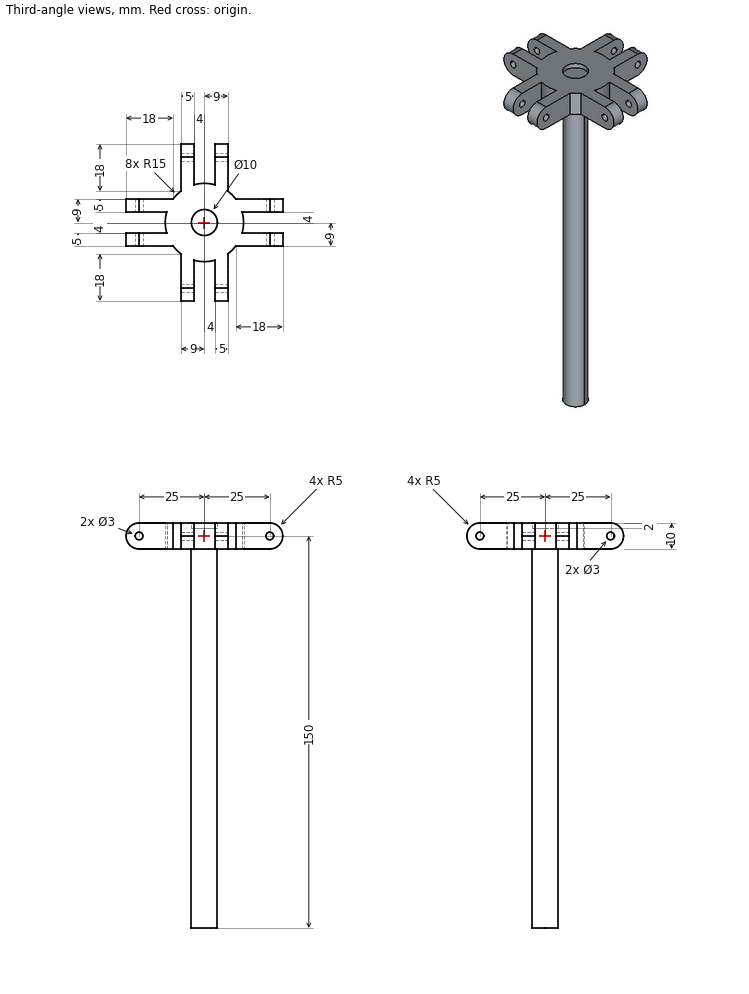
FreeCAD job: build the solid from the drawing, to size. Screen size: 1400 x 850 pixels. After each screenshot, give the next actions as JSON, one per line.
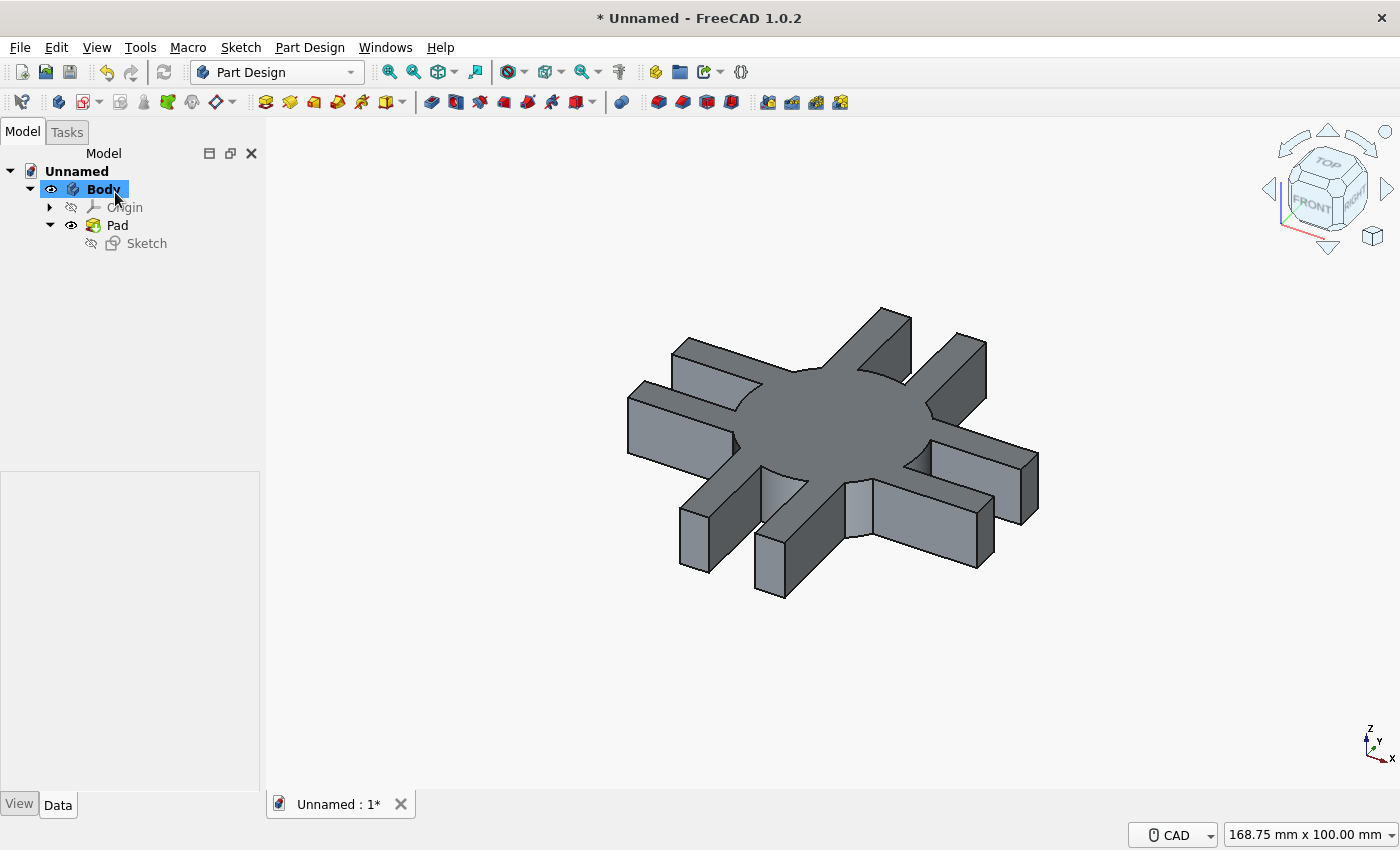
{"action": "left_click", "coordinate": [84, 102]}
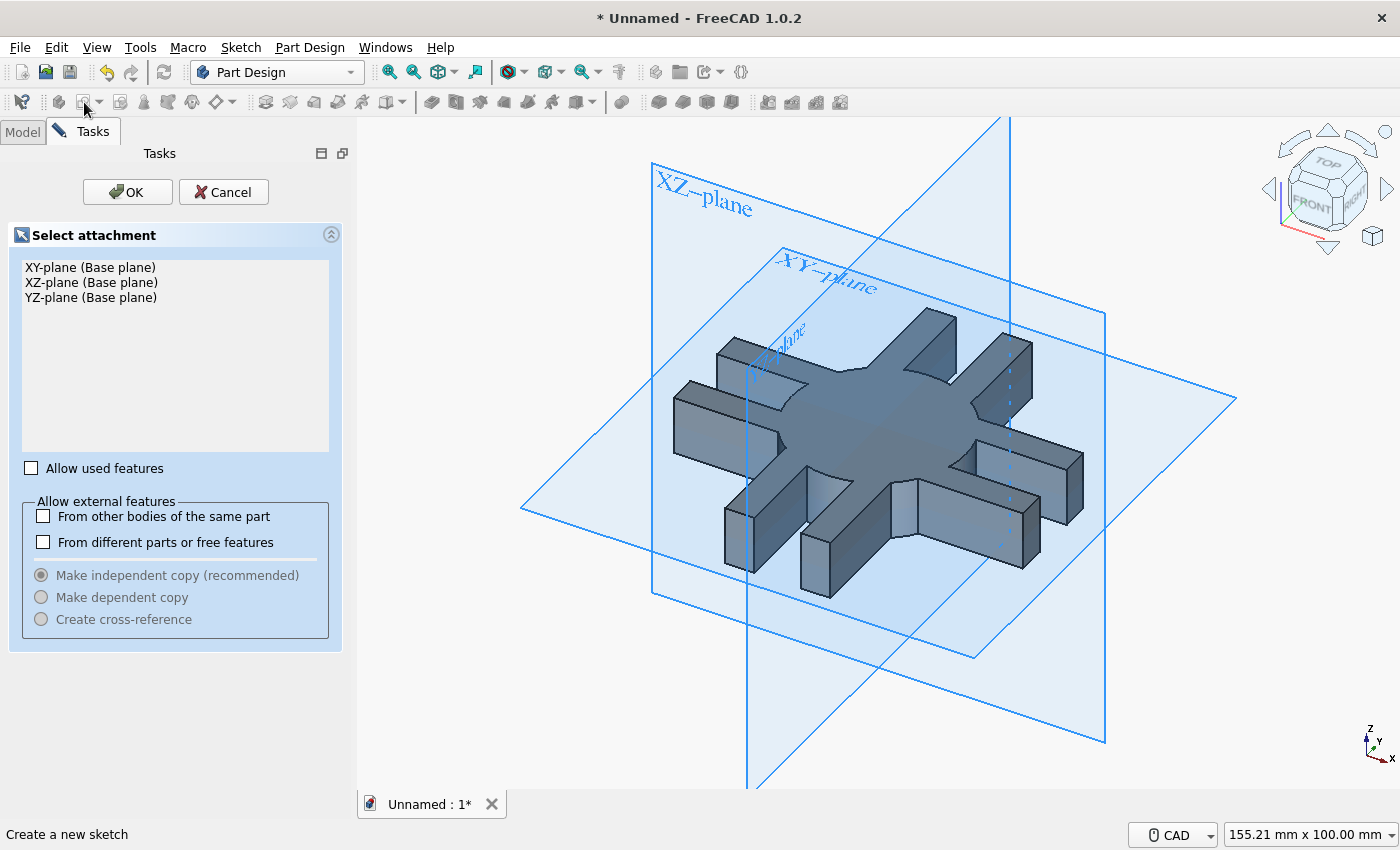
{"action": "left_click", "coordinate": [82, 268]}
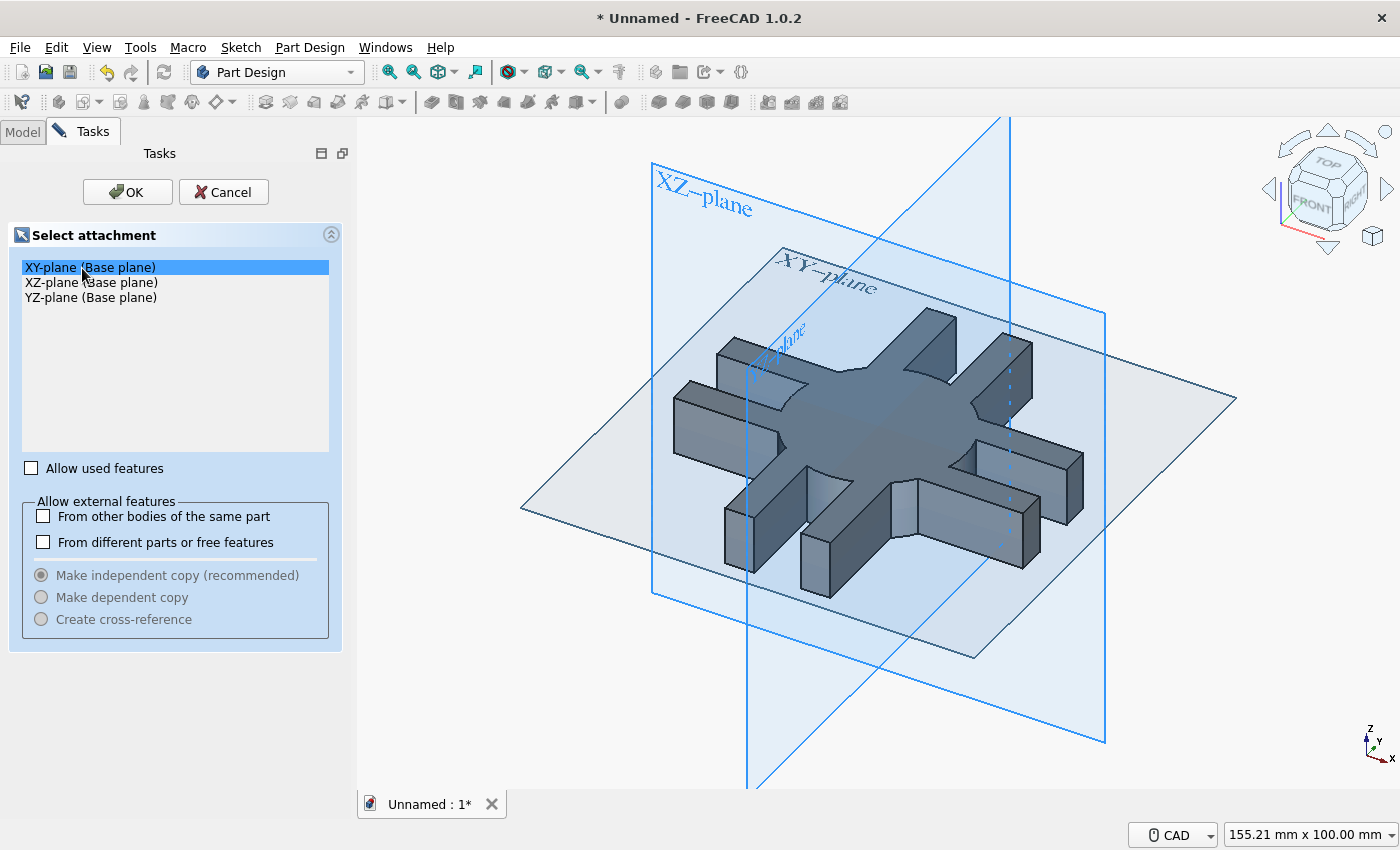
{"action": "left_click", "coordinate": [128, 192]}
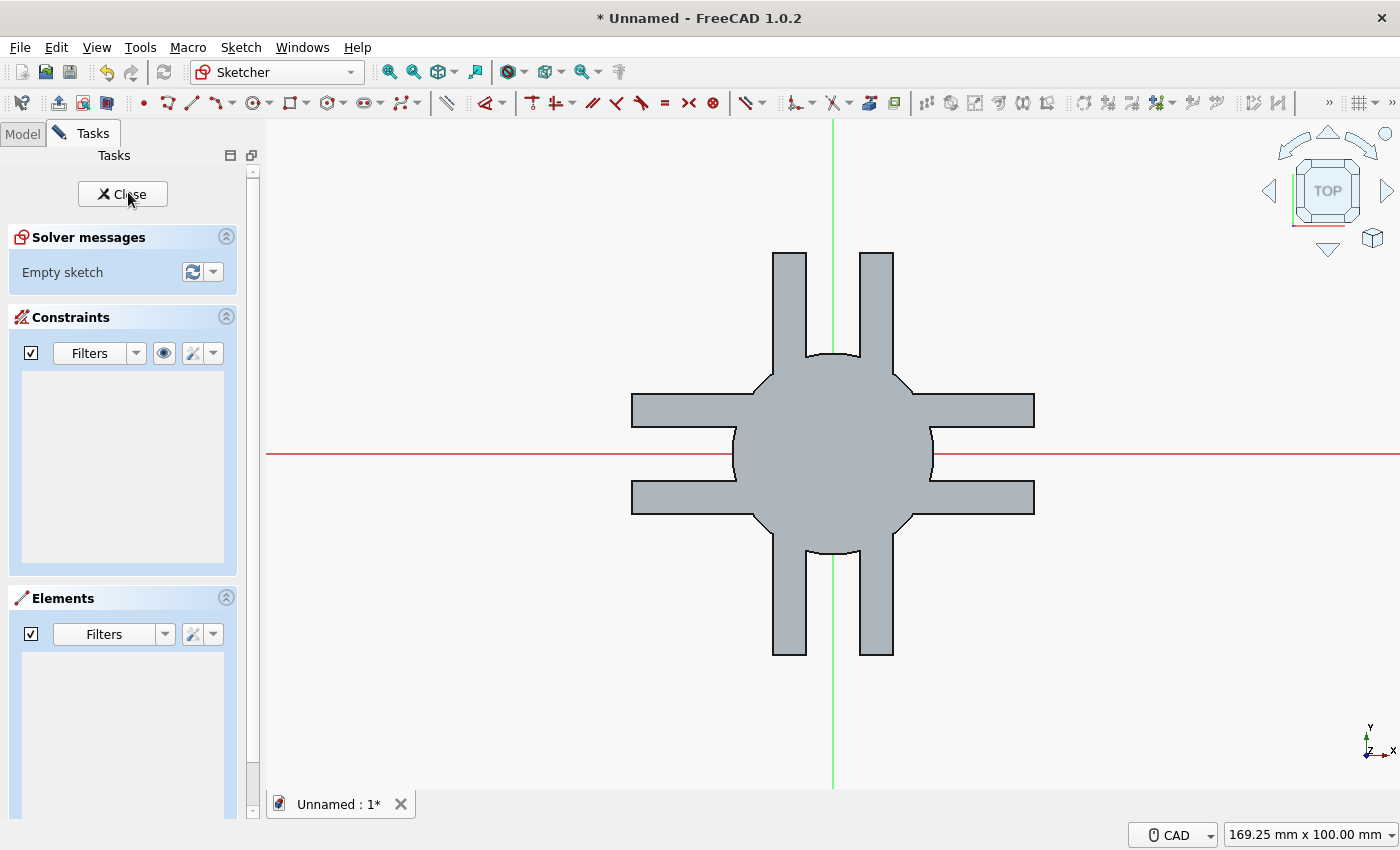
{"action": "left_click", "coordinate": [108, 104]}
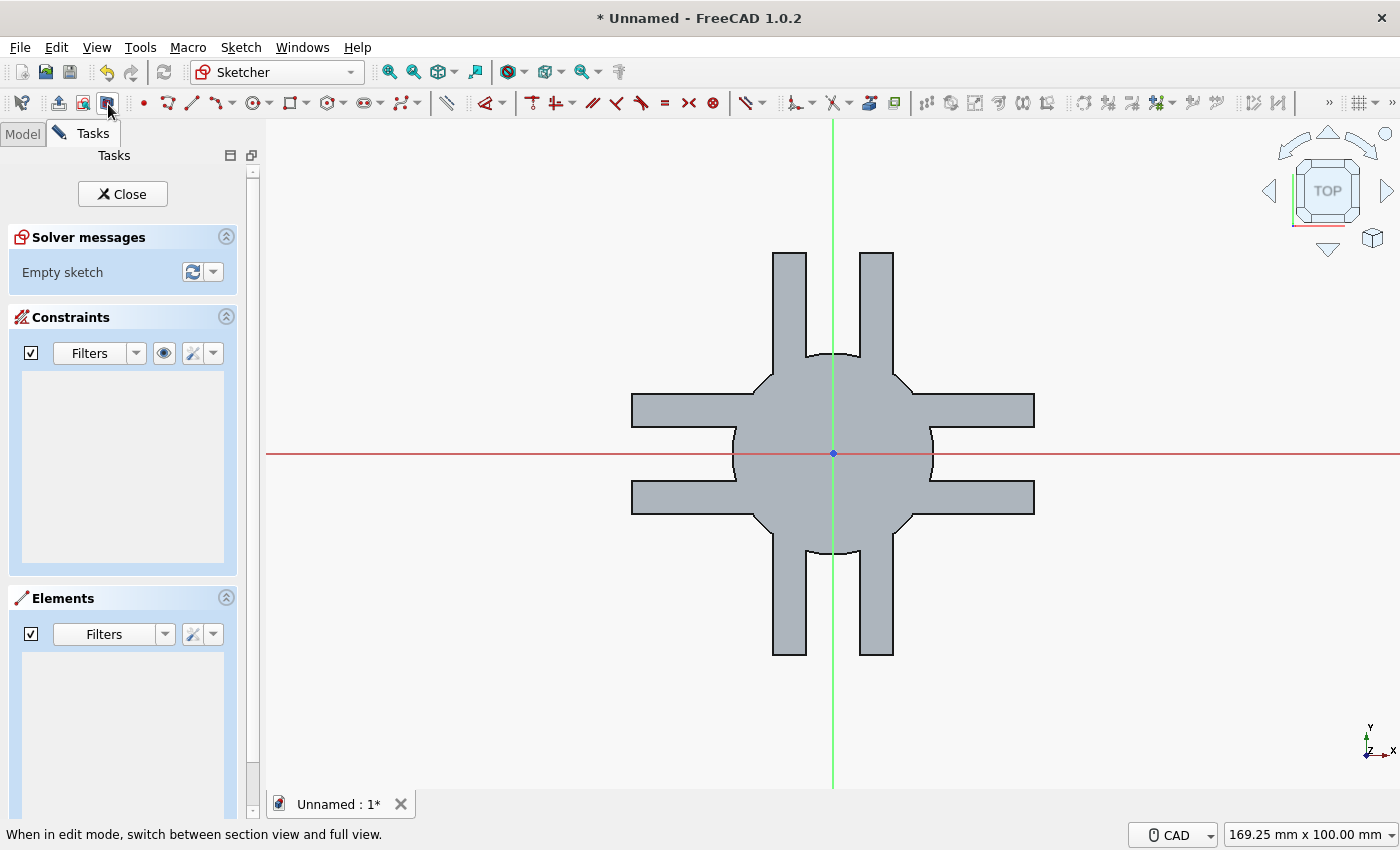
{"action": "scroll", "coordinate": [847, 454], "scroll_direction": "up", "scroll_amount": 9}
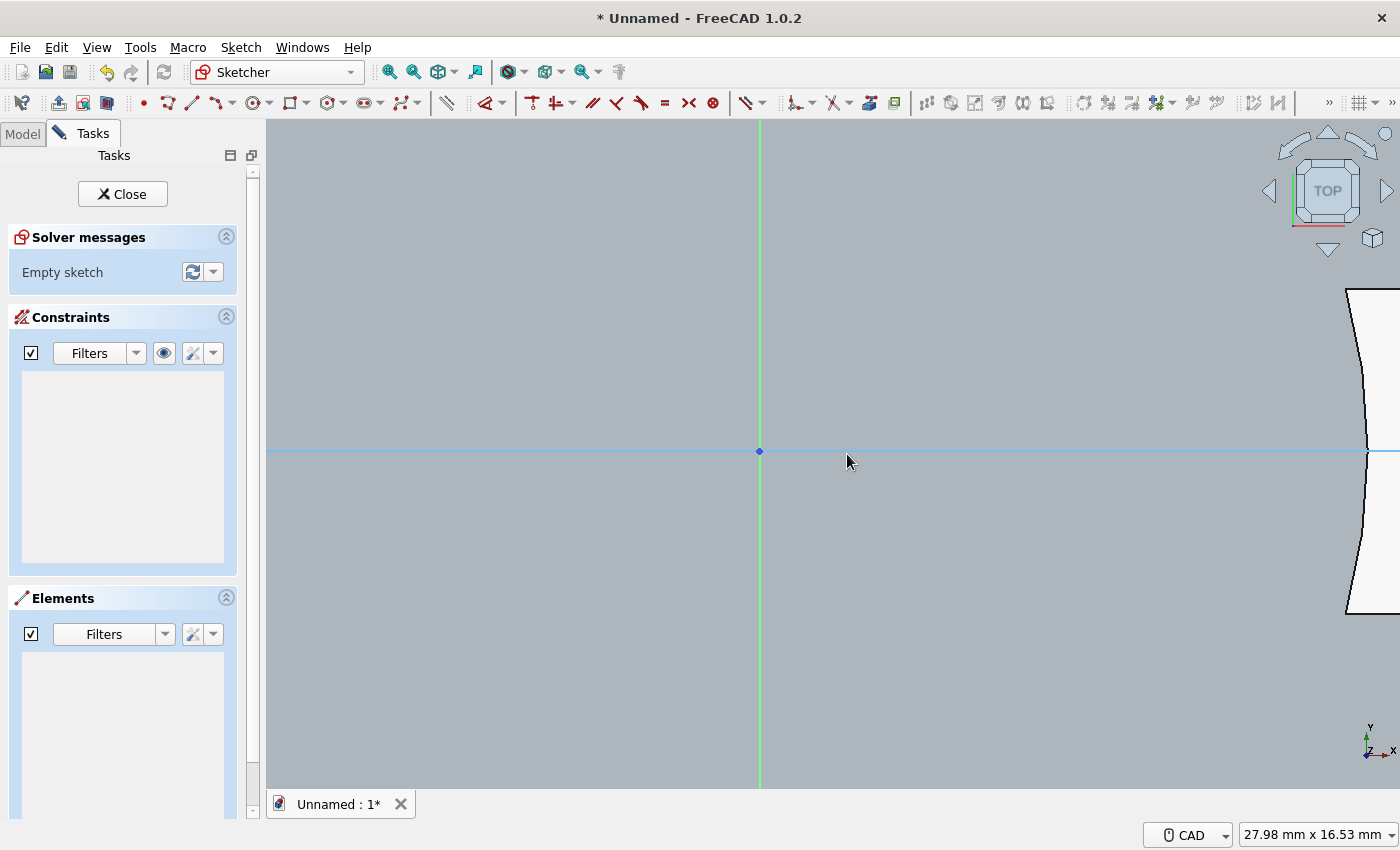
{"action": "left_click", "coordinate": [254, 104]}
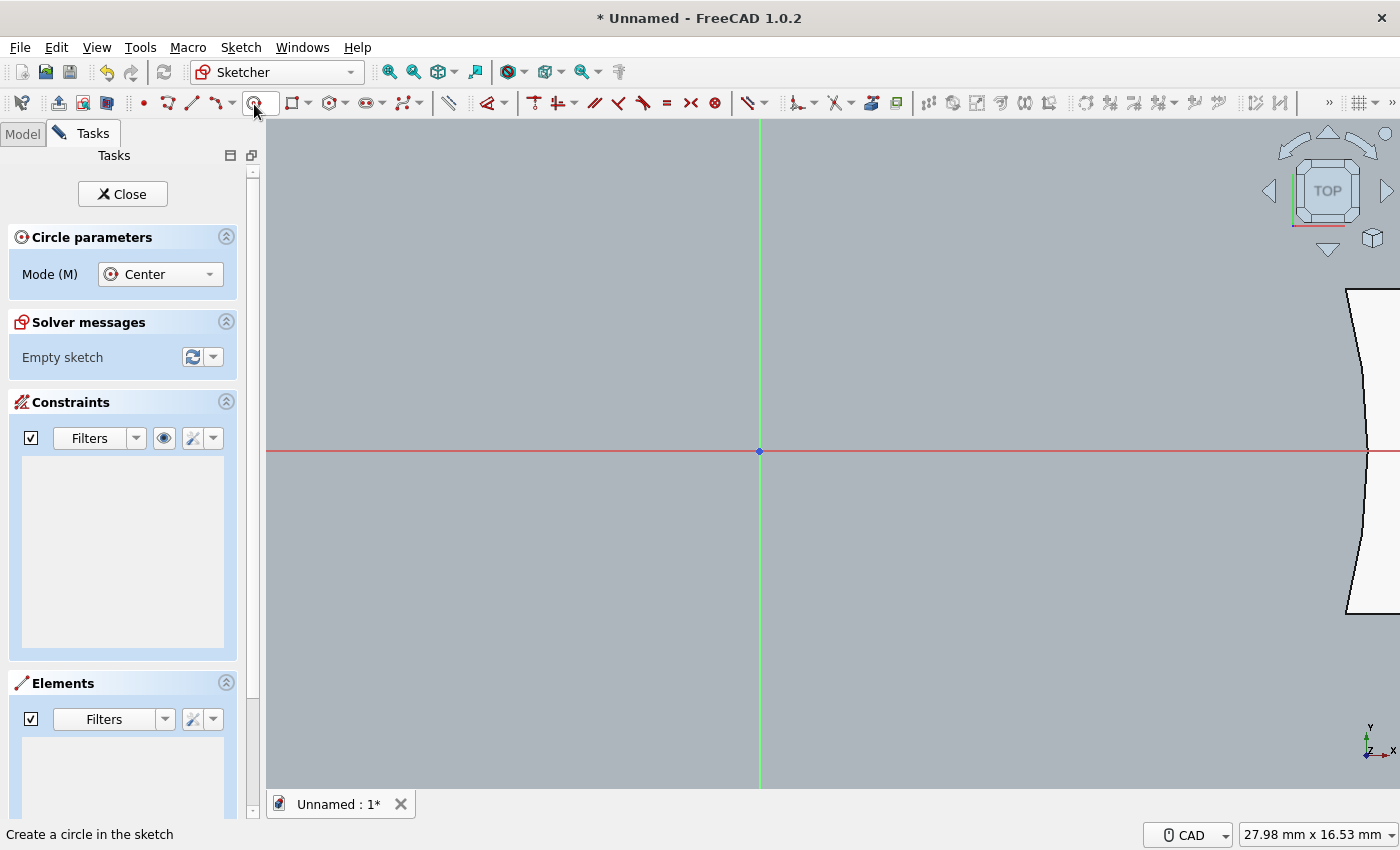
{"action": "left_click", "coordinate": [760, 451]}
{"action": "mouse_move", "coordinate": [903, 308]}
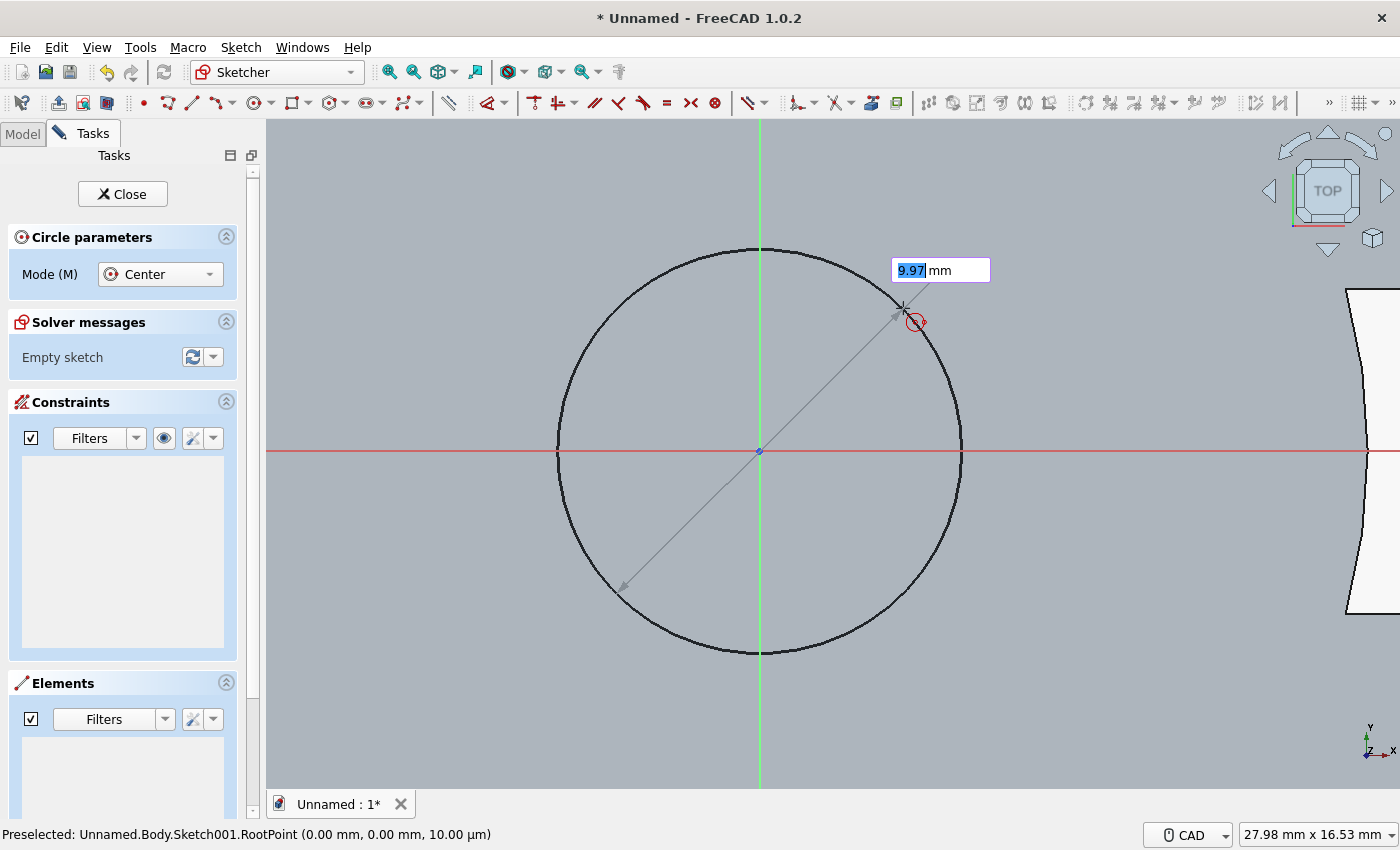
{"action": "type", "text": "10"}
{"action": "key", "text": "Return"}
{"action": "key", "text": "Escape"}